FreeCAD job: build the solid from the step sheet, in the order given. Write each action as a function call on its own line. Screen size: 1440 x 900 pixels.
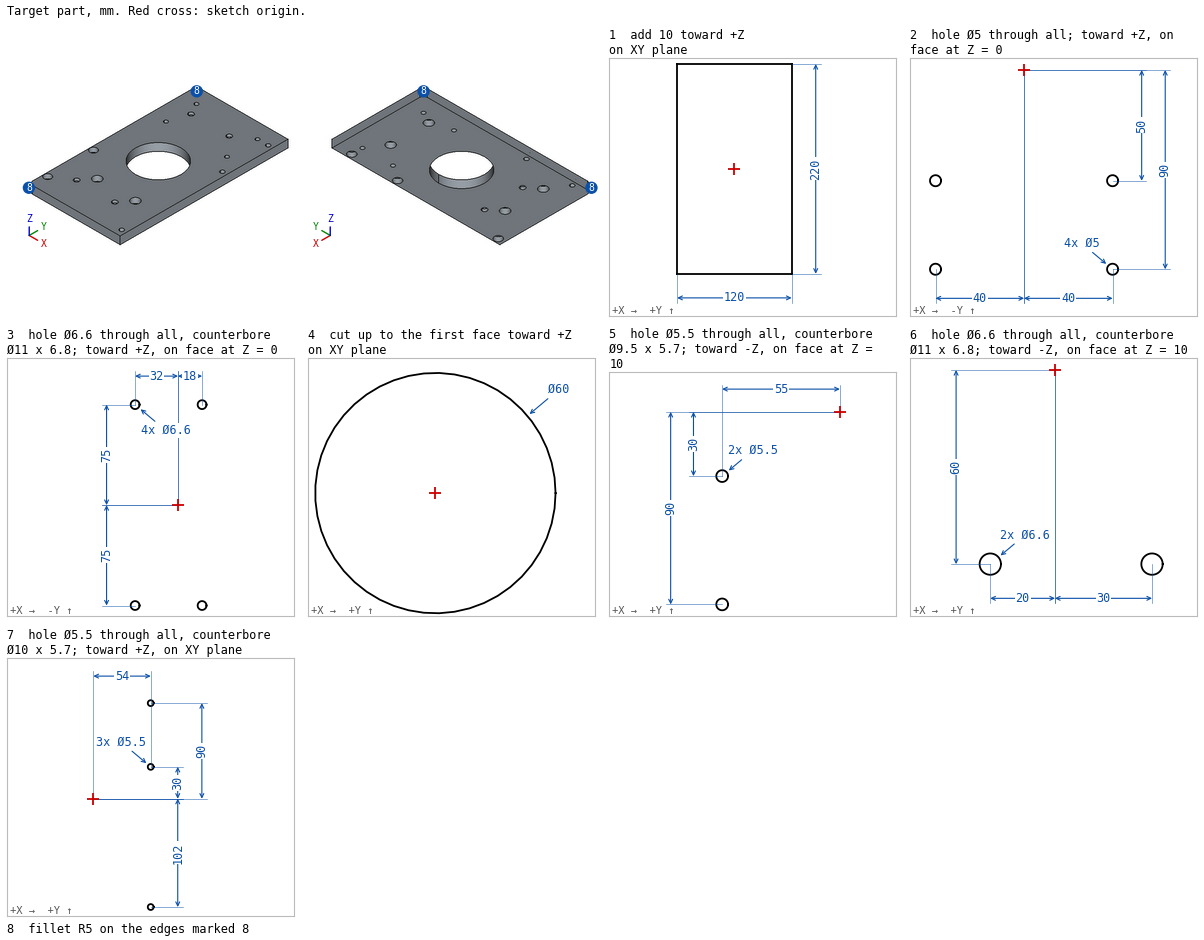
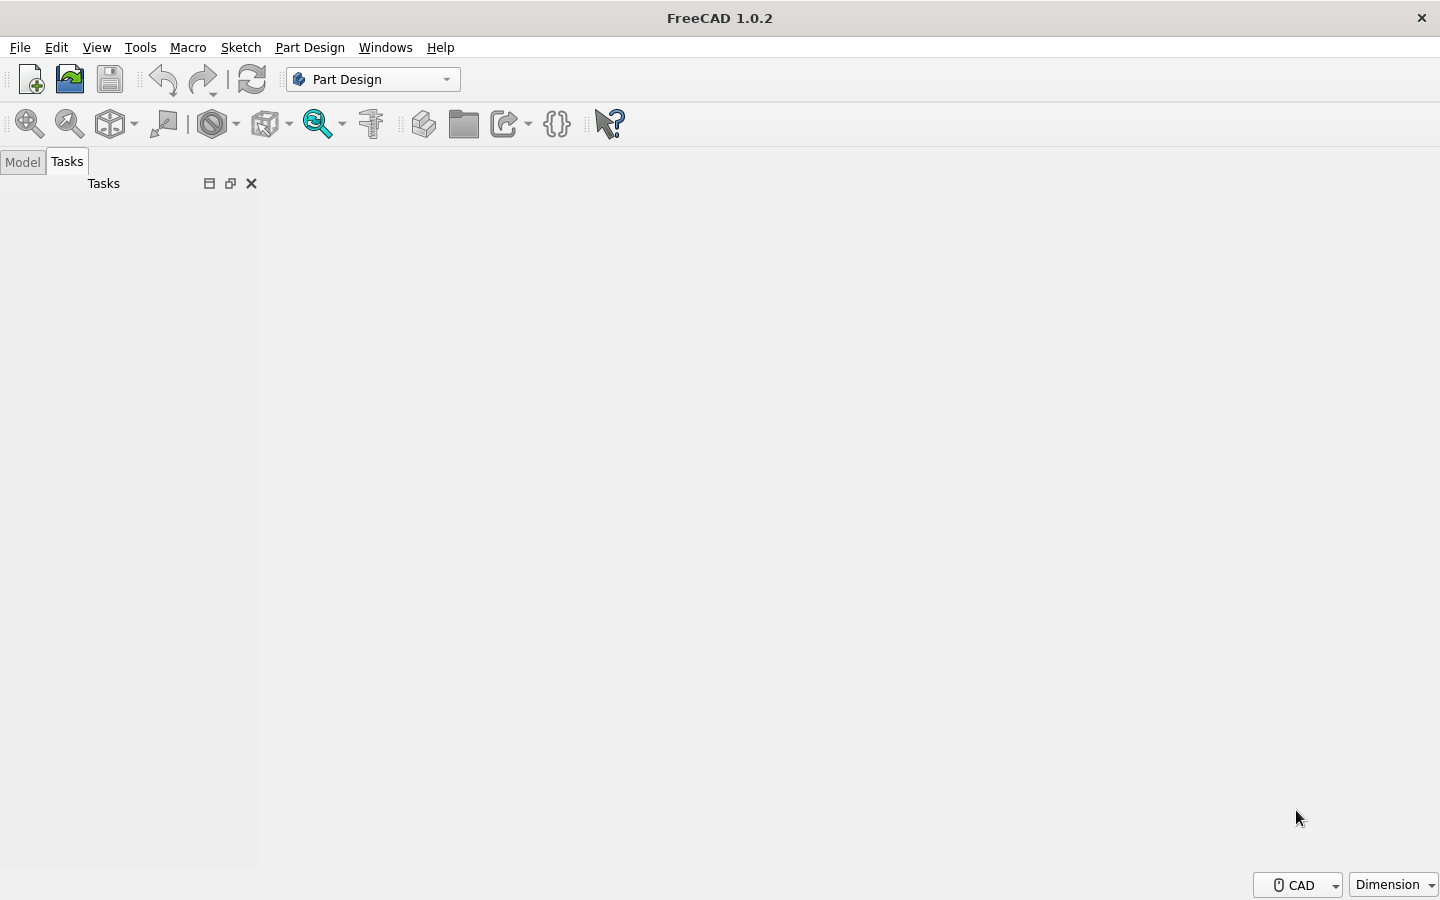
key(ctrl+n)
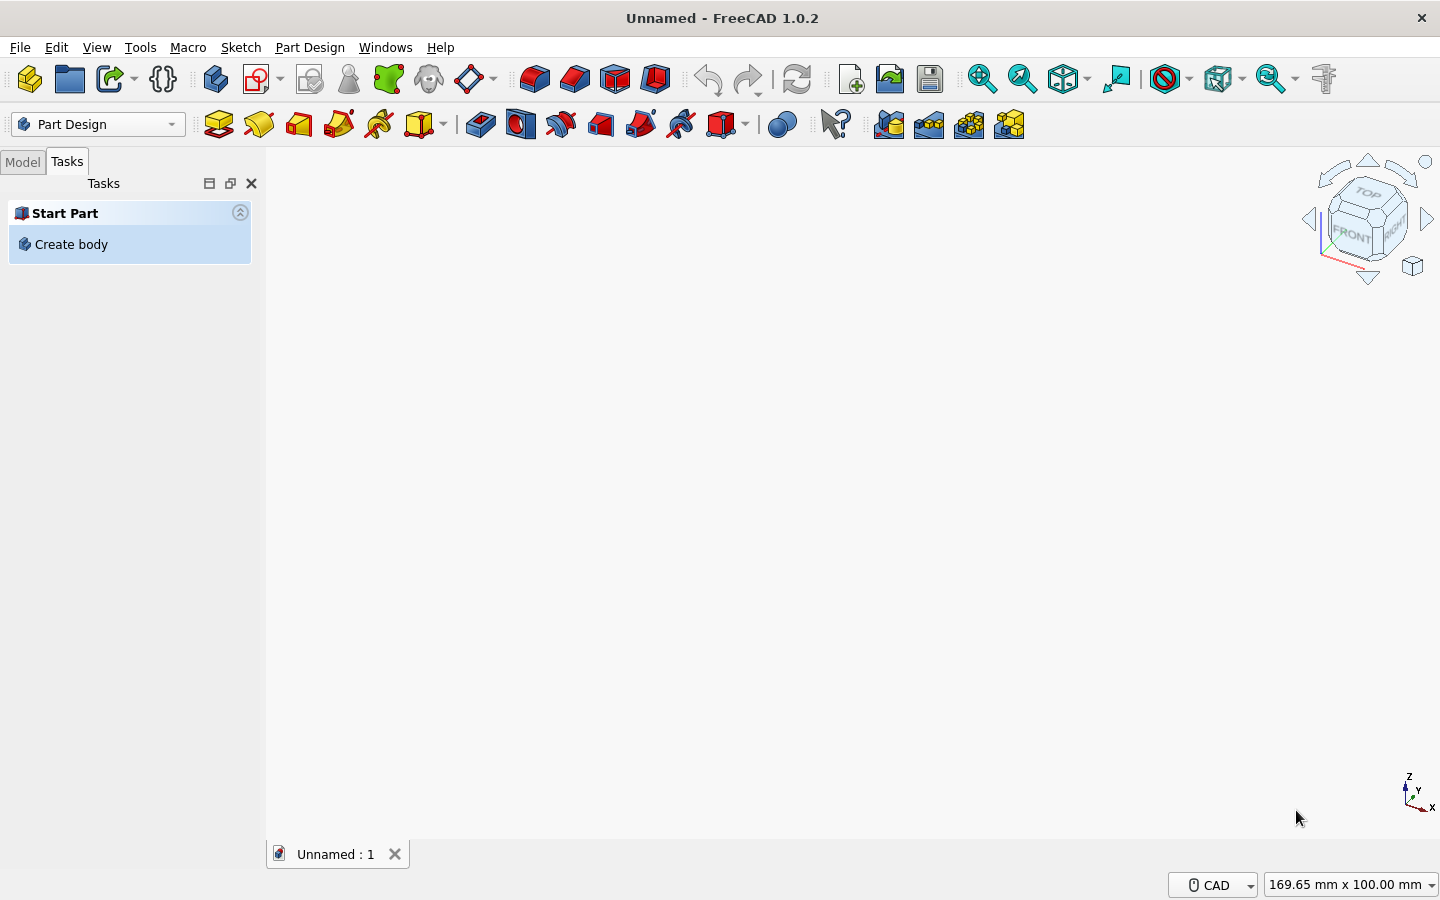
click(256, 80)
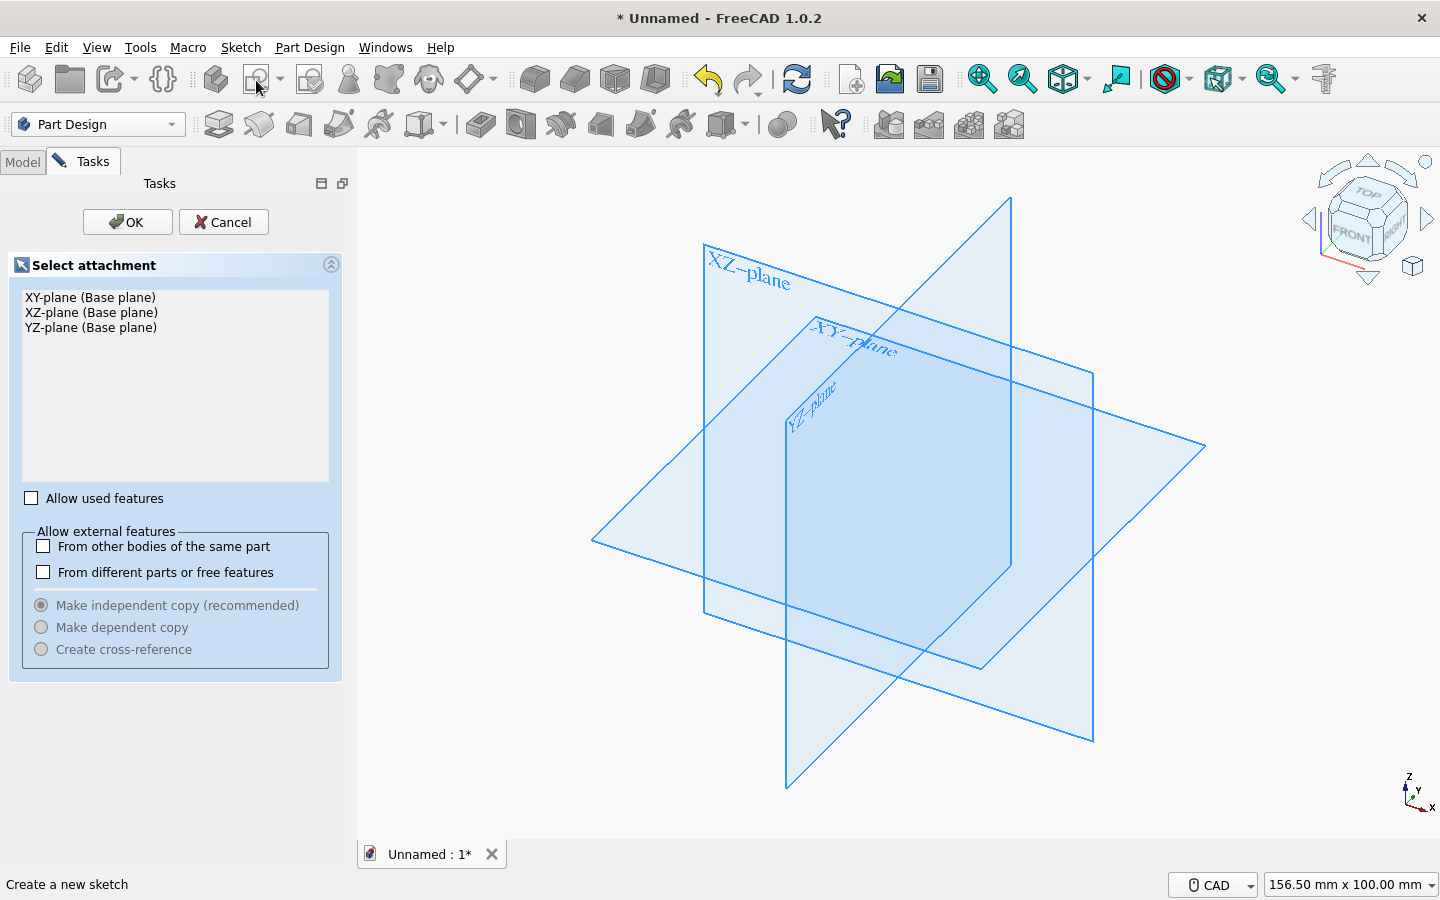
click(82, 298)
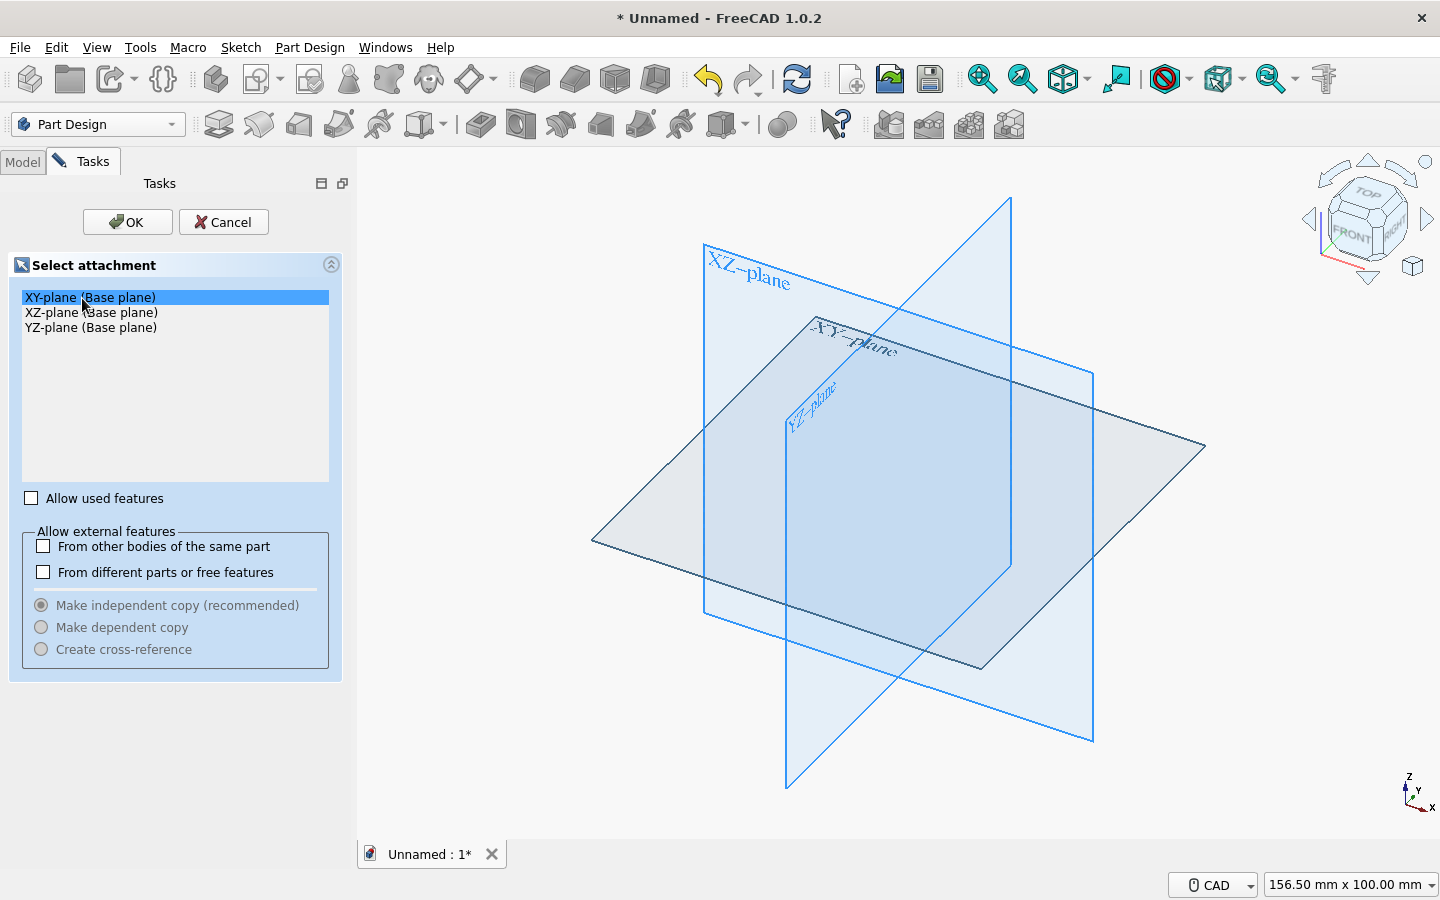
click(128, 222)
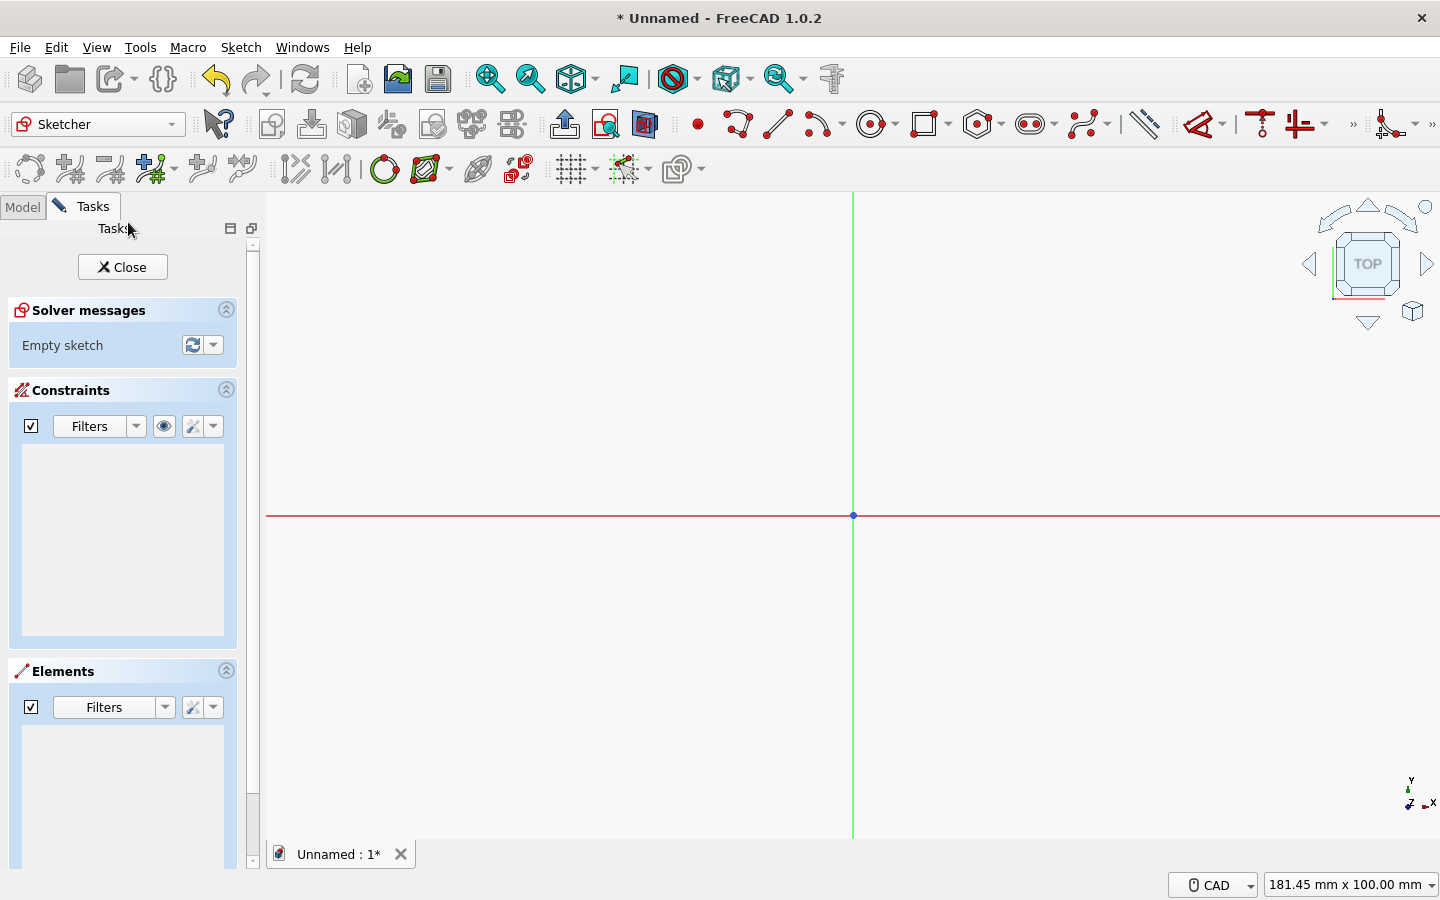
scroll(755, 516, down, 6)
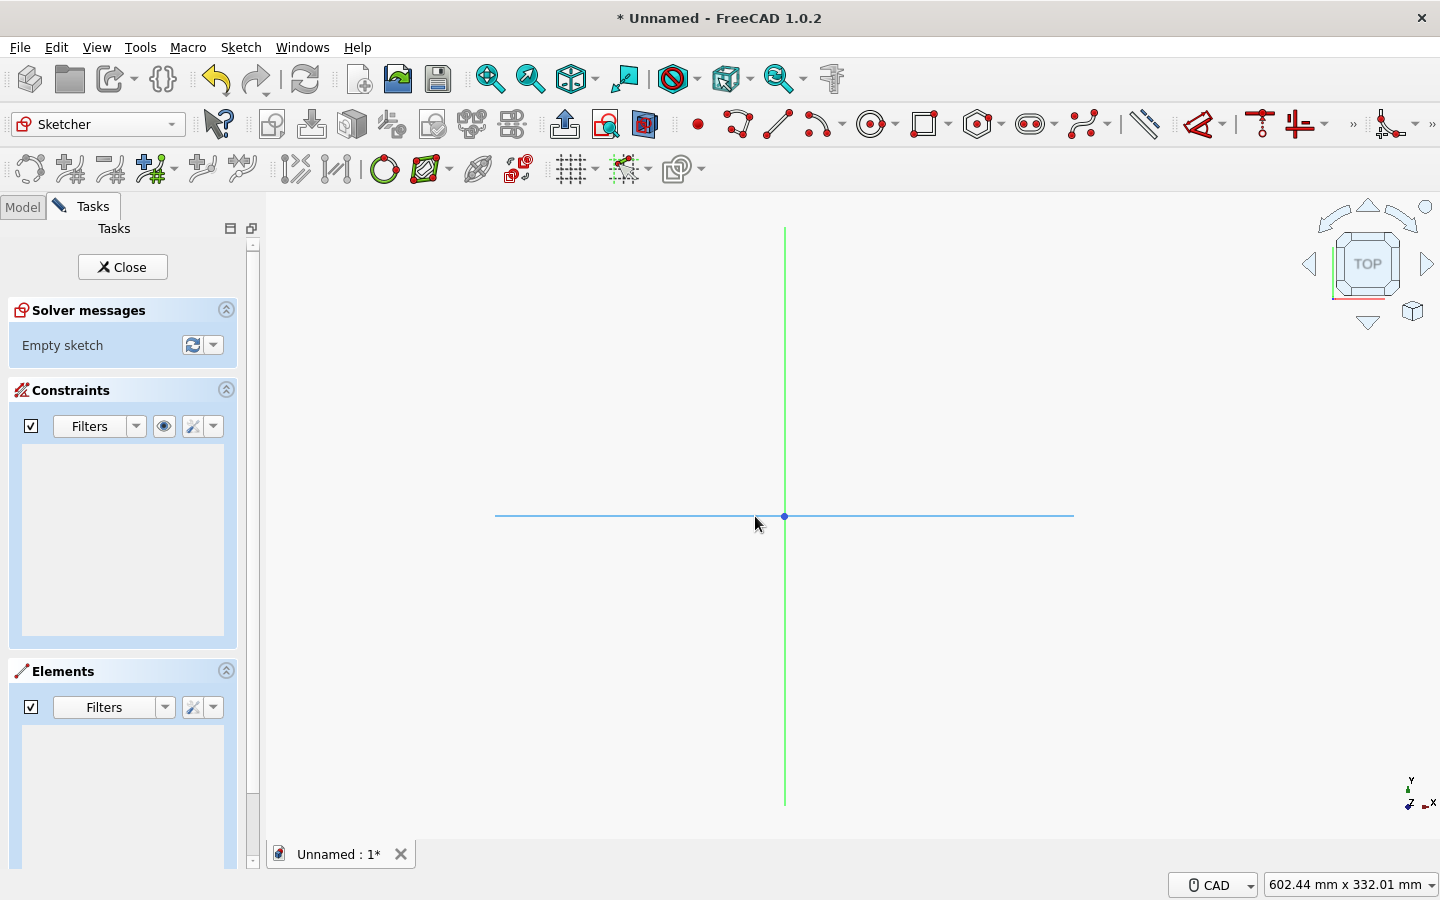
key(g)
key(v)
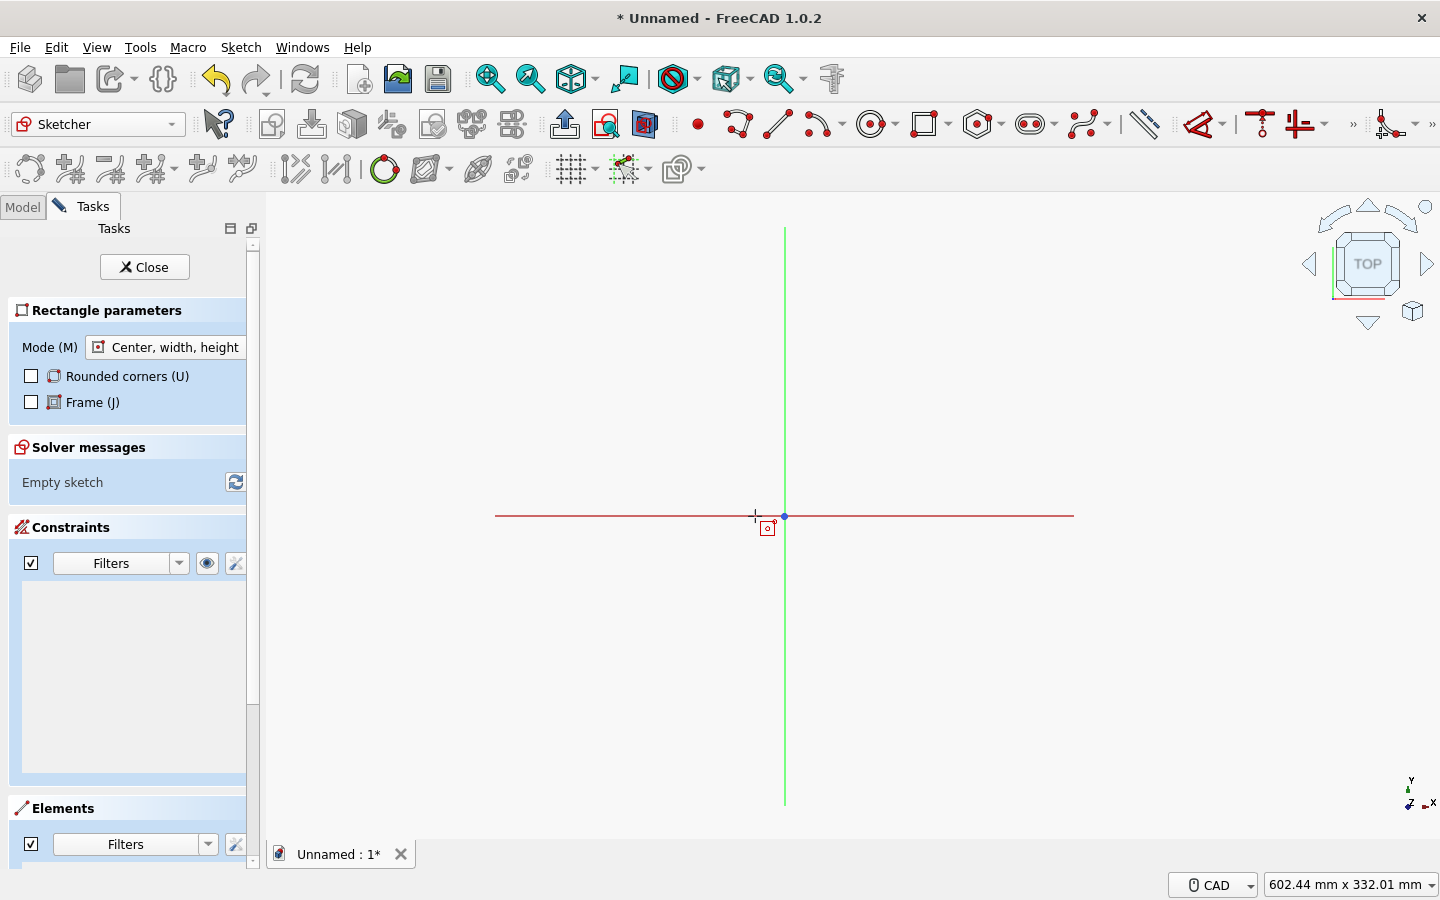
click(785, 516)
move(902, 302)